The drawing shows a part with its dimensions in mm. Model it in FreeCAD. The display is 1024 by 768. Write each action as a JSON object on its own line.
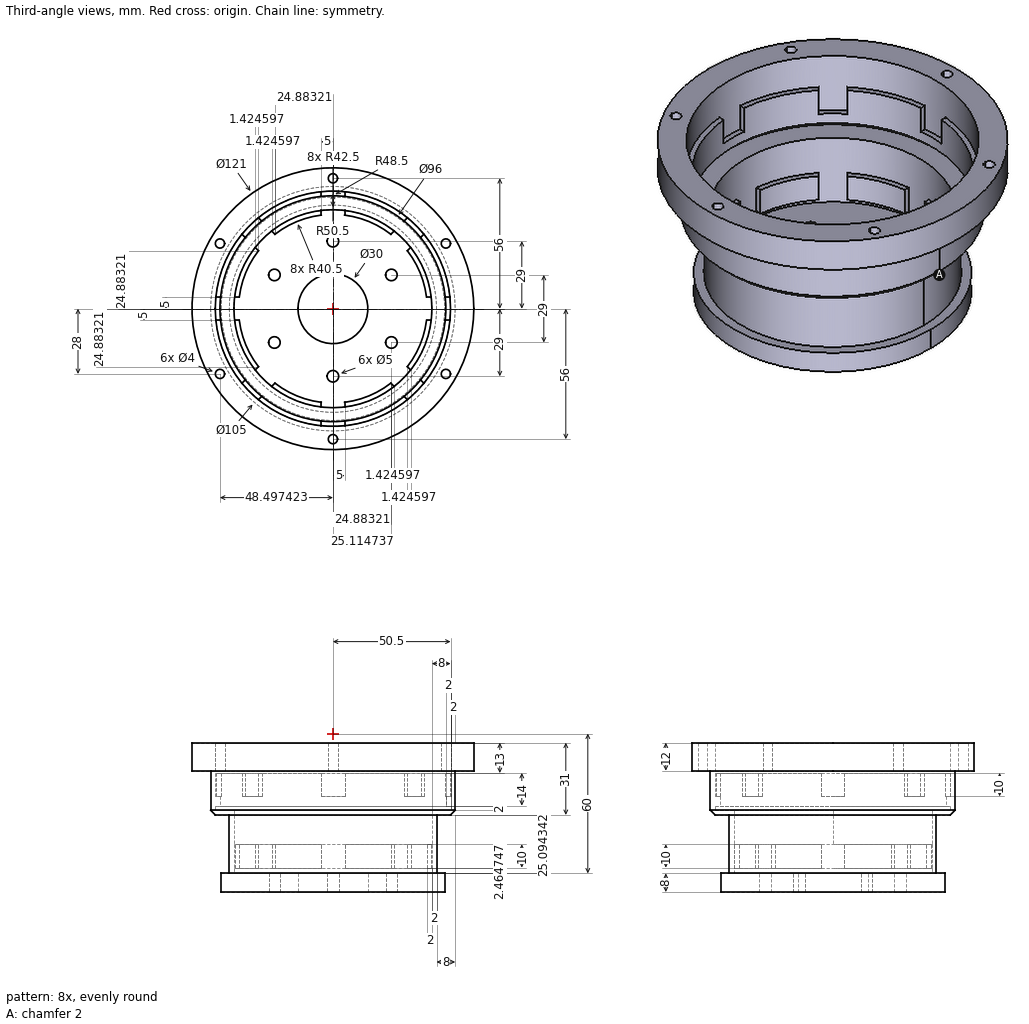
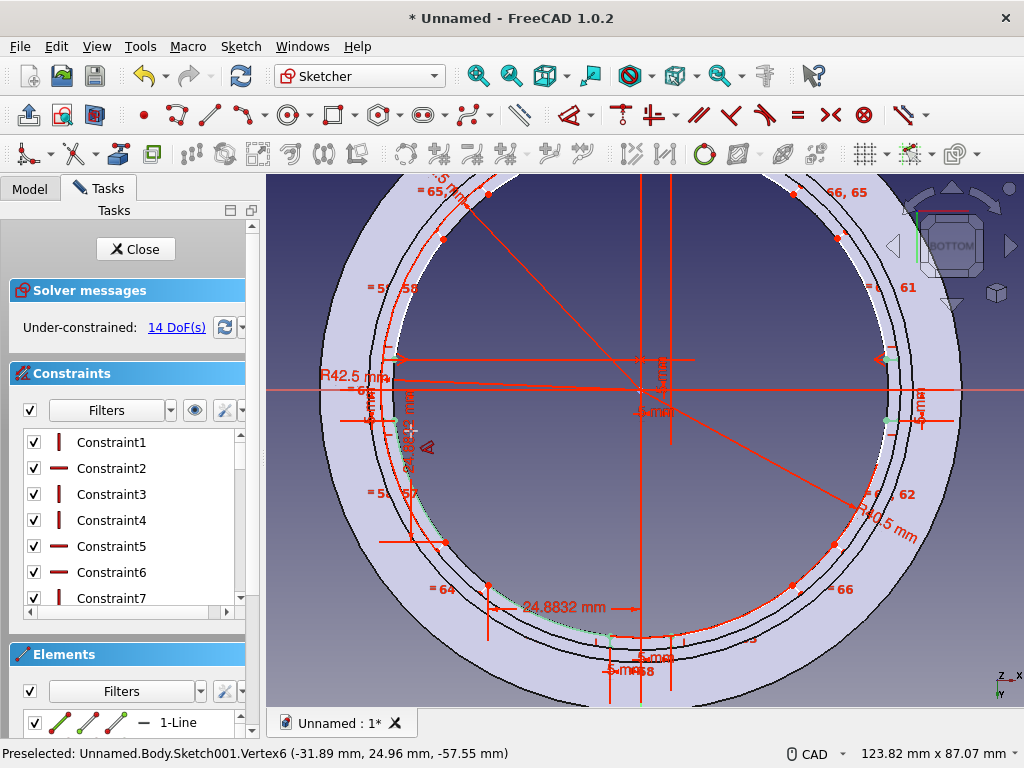
{"action": "left_click", "coordinate": [444, 239]}
{"action": "left_click", "coordinate": [410, 349]}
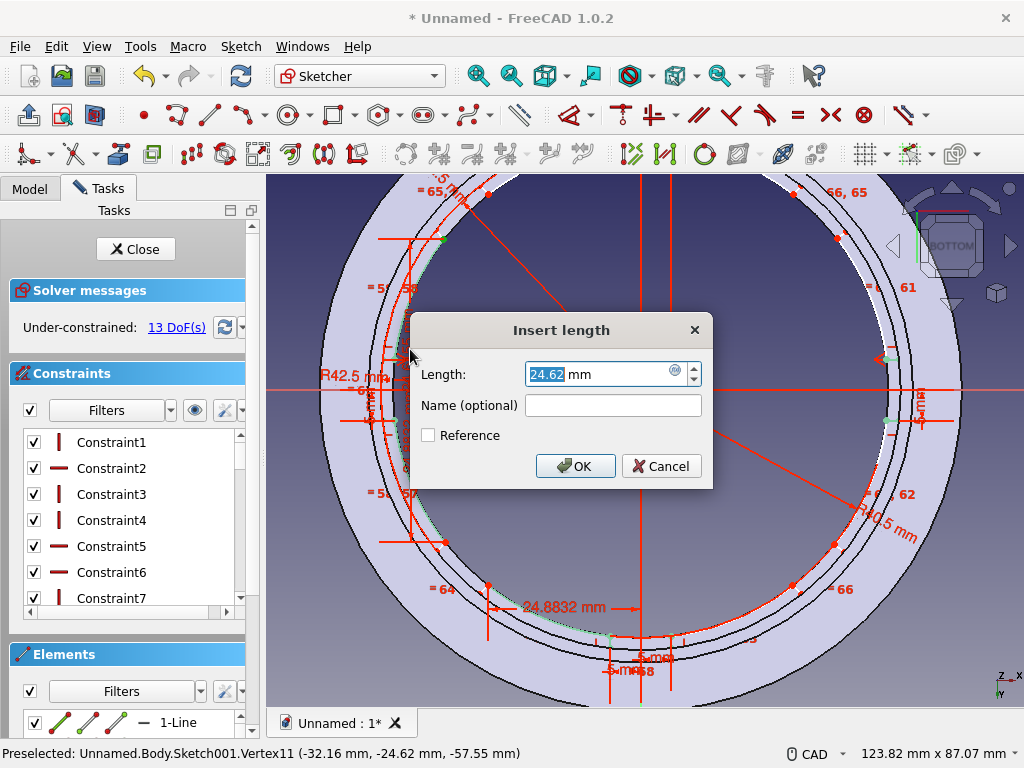
{"action": "type", "text": "24.88321"}
{"action": "key", "text": "Return"}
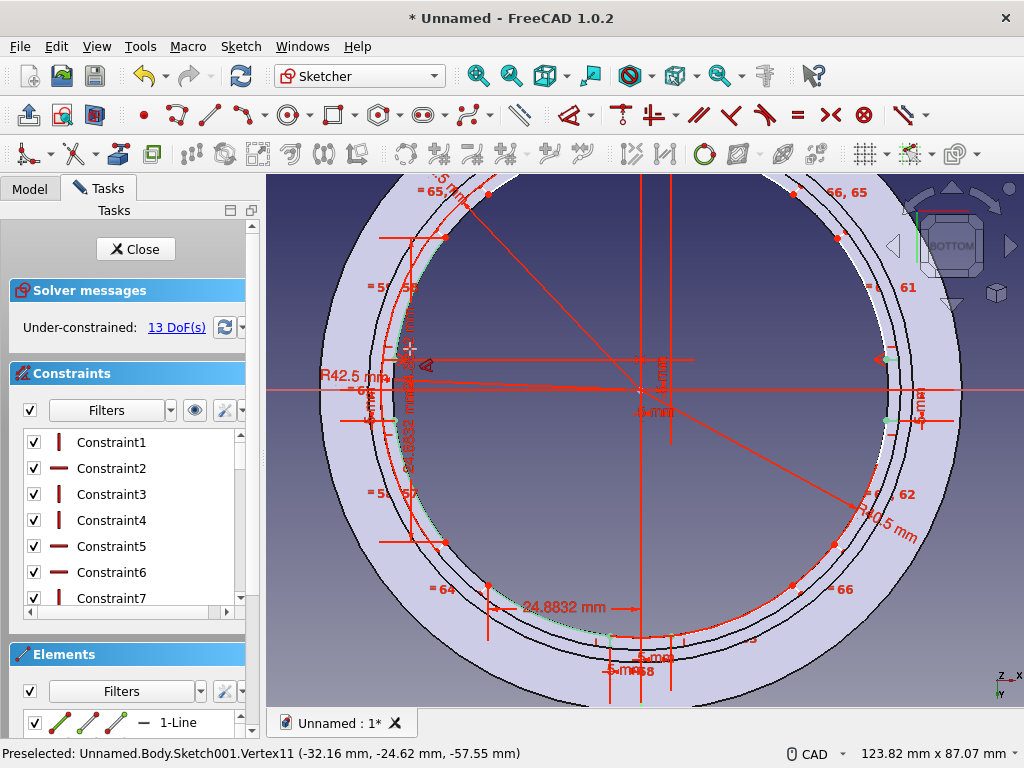
{"action": "scroll", "coordinate": [446, 543], "scroll_direction": "down", "scroll_amount": 2}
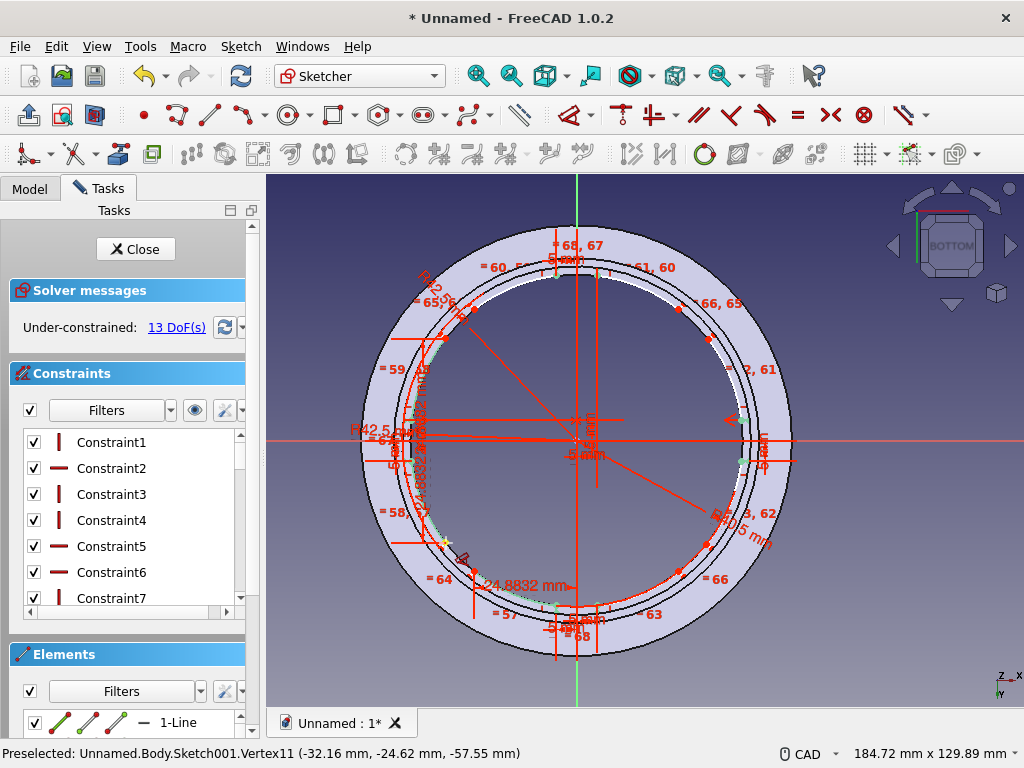
{"action": "scroll", "coordinate": [475, 310], "scroll_direction": "up", "scroll_amount": 2}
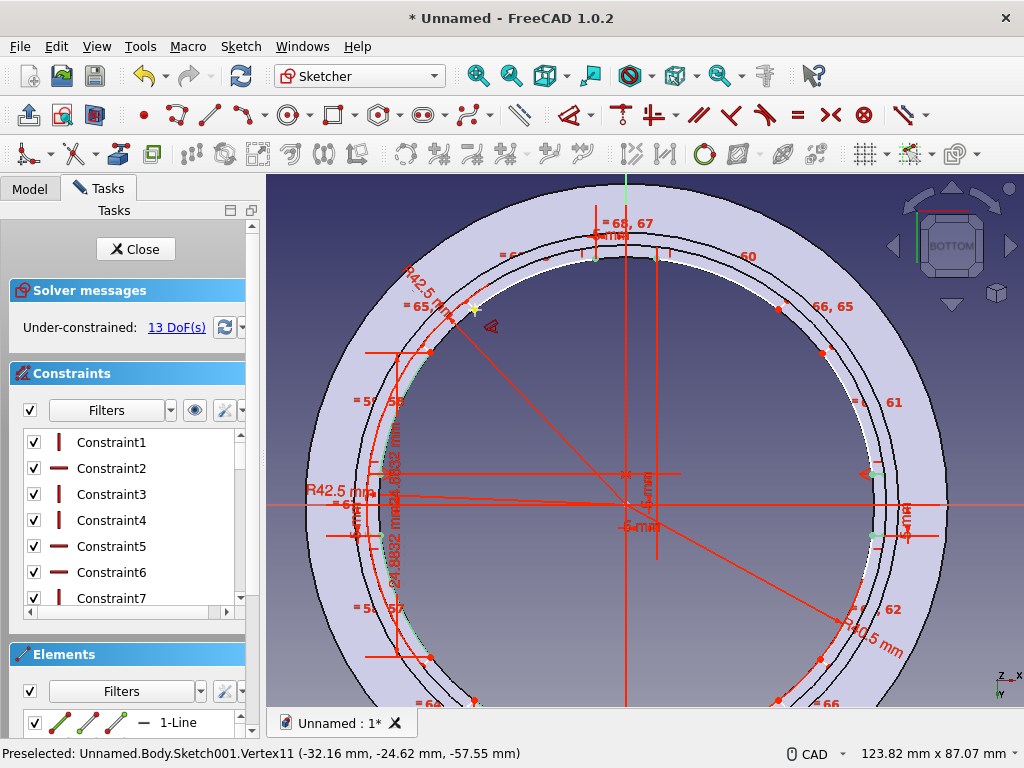
{"action": "left_click", "coordinate": [474, 309]}
{"action": "left_click", "coordinate": [585, 275]}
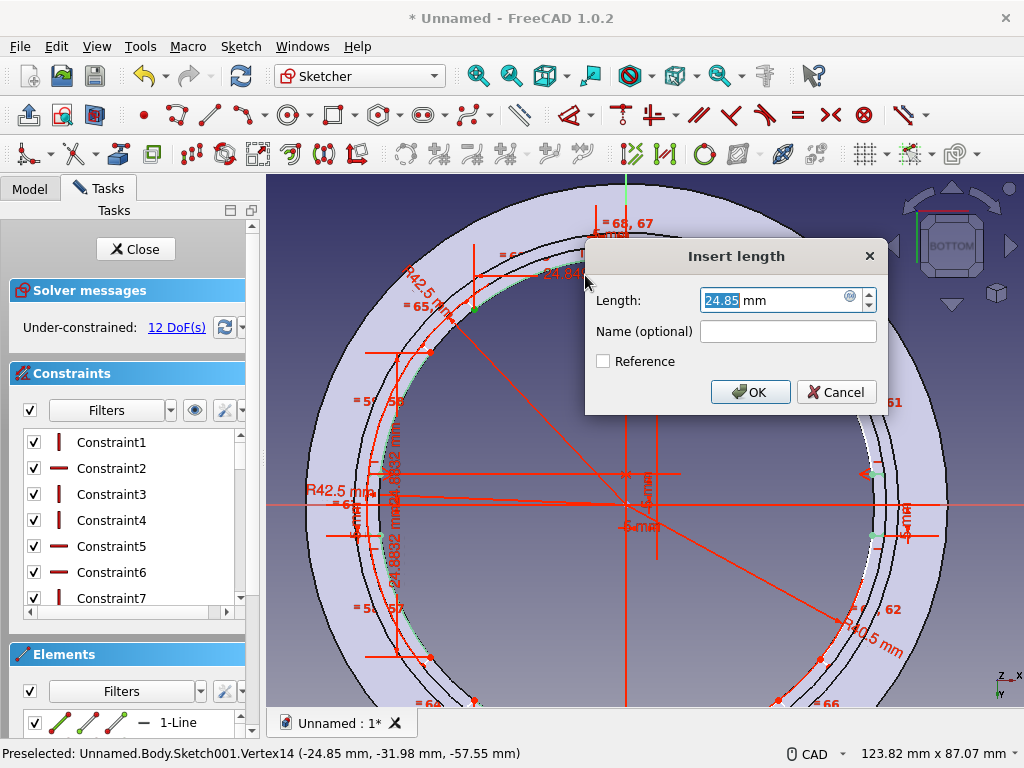
{"action": "type", "text": "24.88321"}
{"action": "key", "text": "Return"}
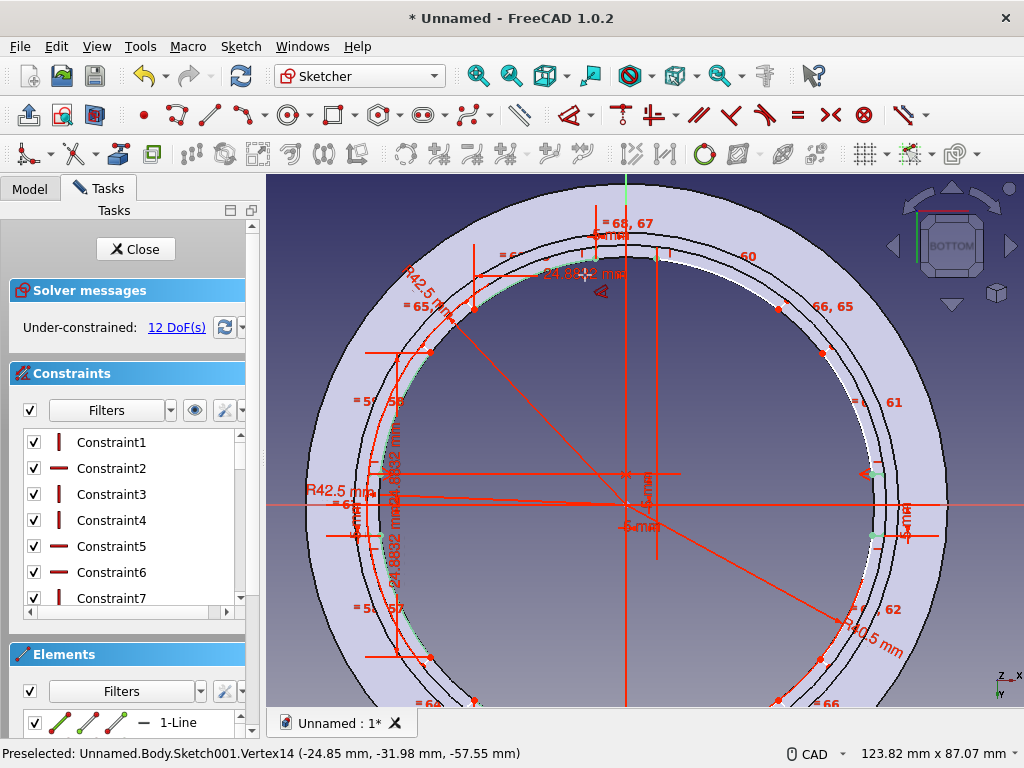
{"action": "left_click", "coordinate": [779, 309]}
{"action": "left_click", "coordinate": [668, 275]}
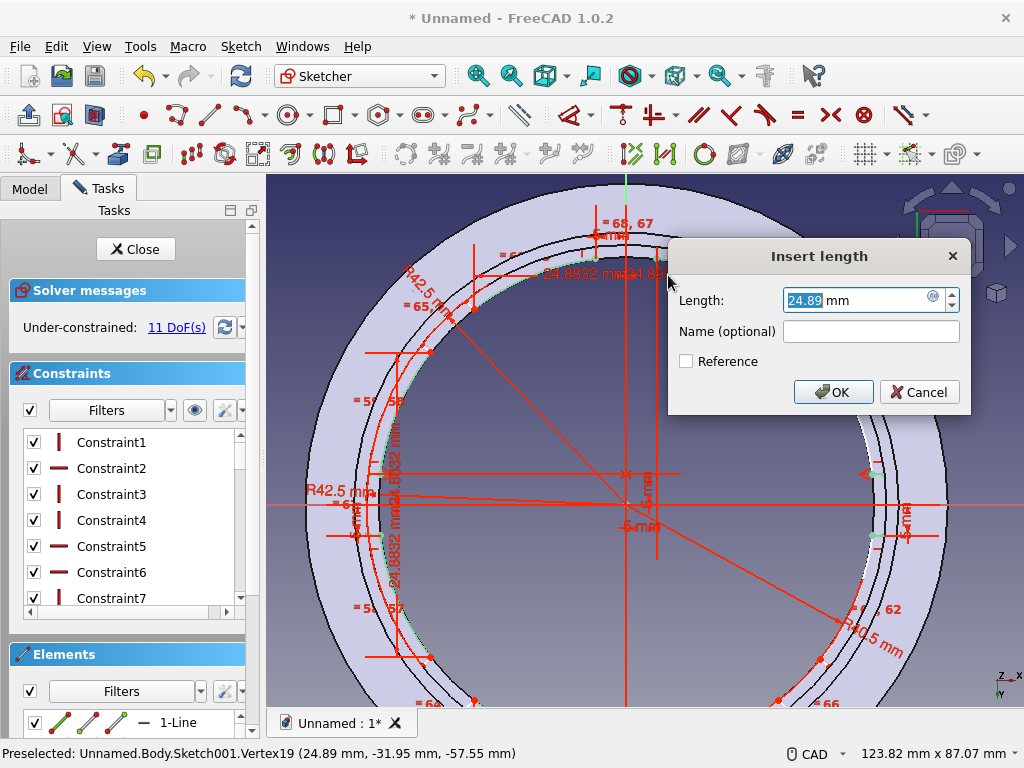
{"action": "type", "text": "24.88321"}
{"action": "key", "text": "Return"}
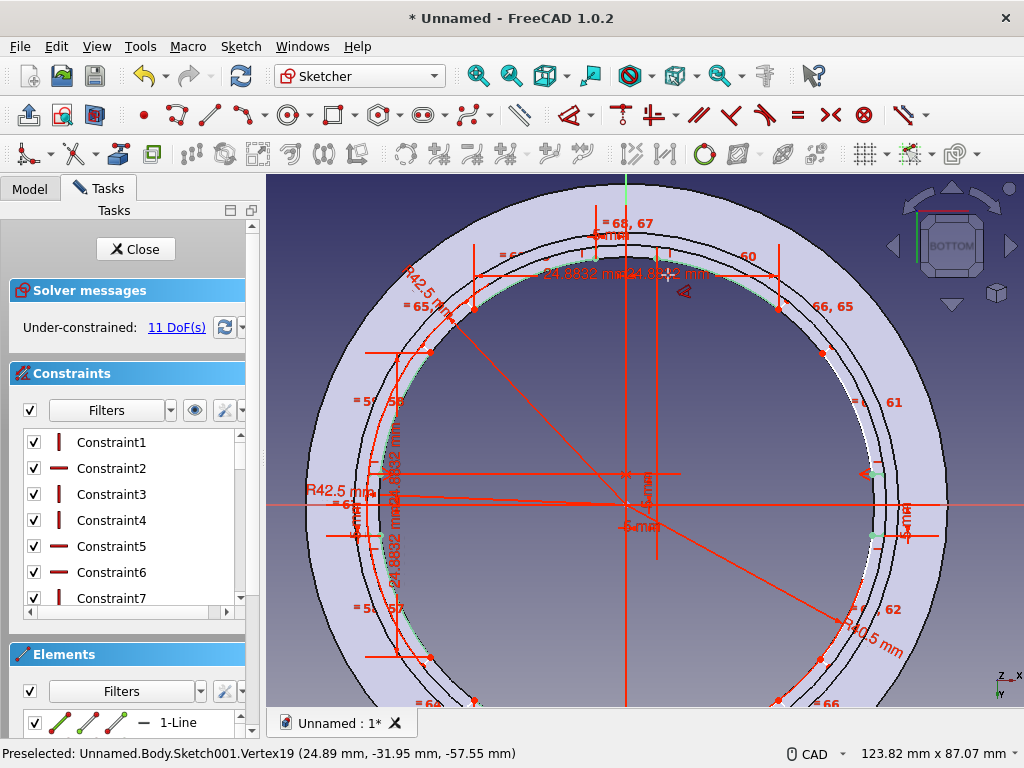
{"action": "left_click", "coordinate": [823, 354]}
{"action": "left_click", "coordinate": [857, 464]}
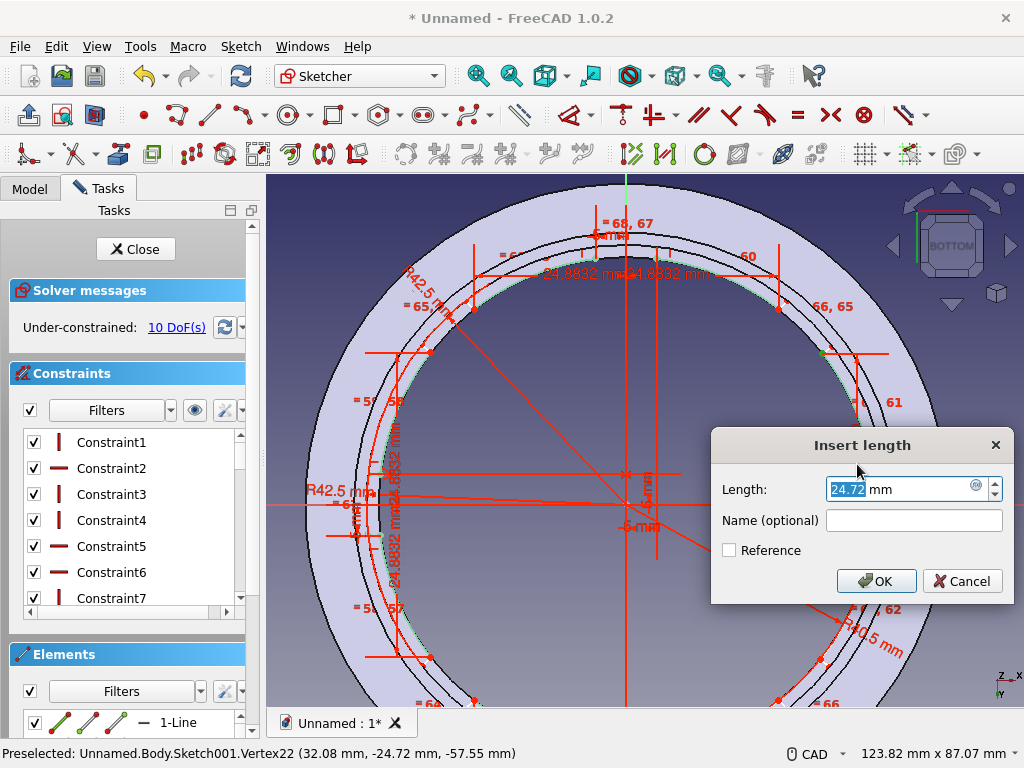
{"action": "type", "text": "24.88321"}
{"action": "key", "text": "Return"}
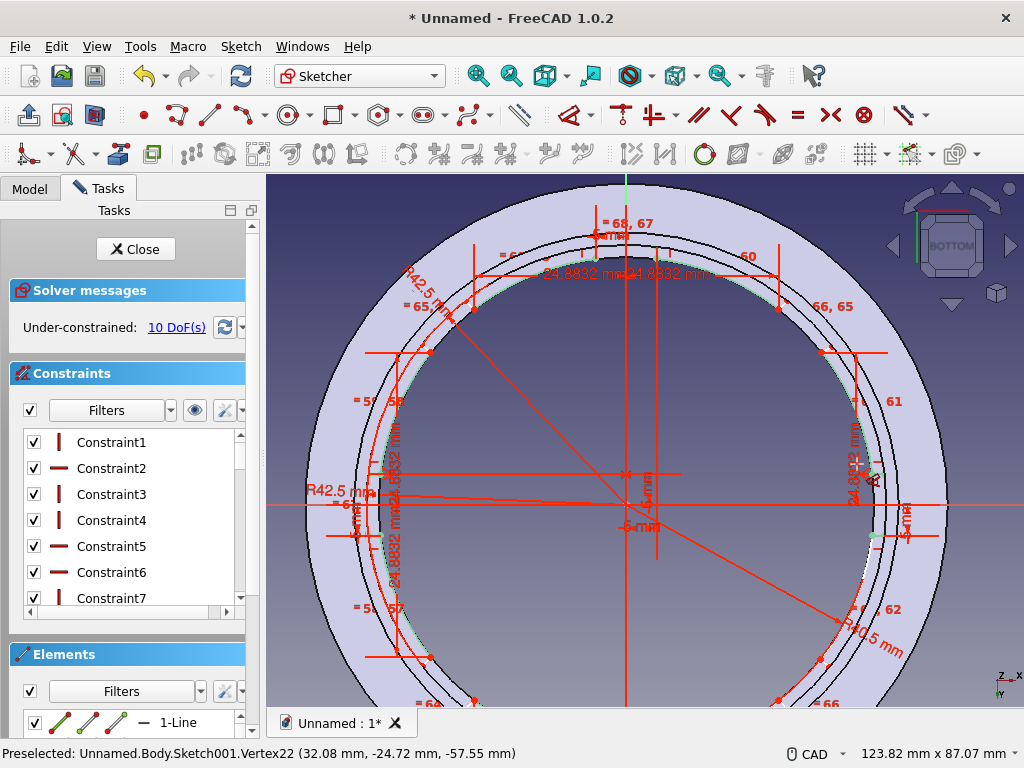
{"action": "left_click", "coordinate": [820, 659]}
{"action": "left_click", "coordinate": [854, 547]}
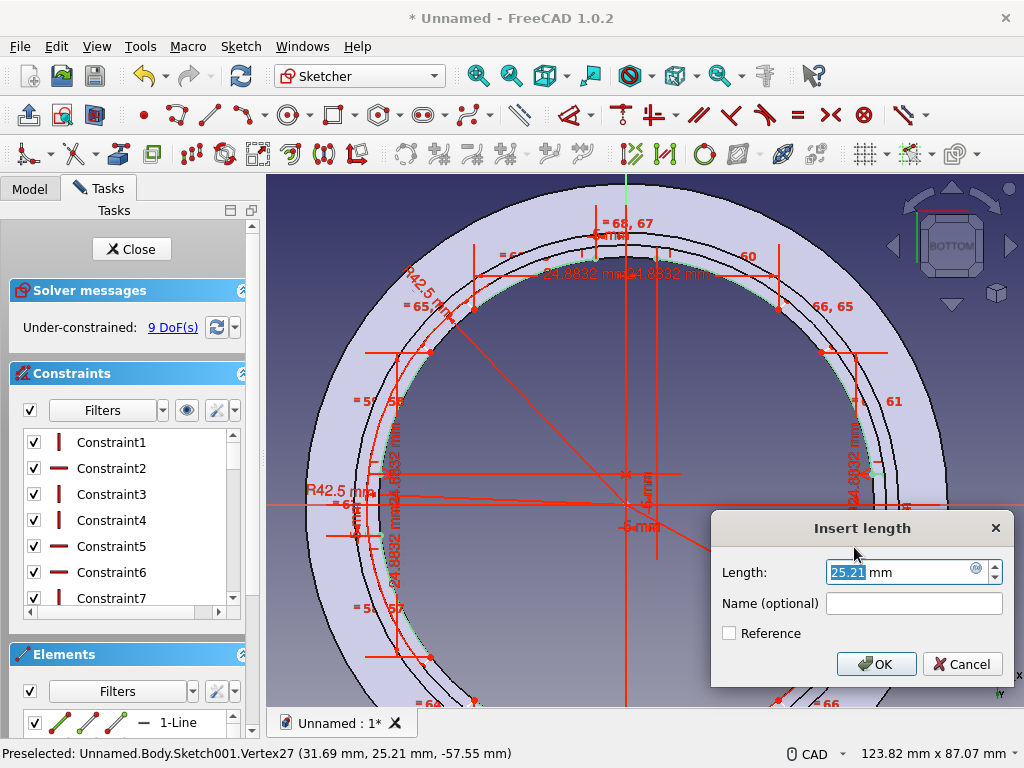
{"action": "type", "text": "24.88321"}
{"action": "key", "text": "Return"}